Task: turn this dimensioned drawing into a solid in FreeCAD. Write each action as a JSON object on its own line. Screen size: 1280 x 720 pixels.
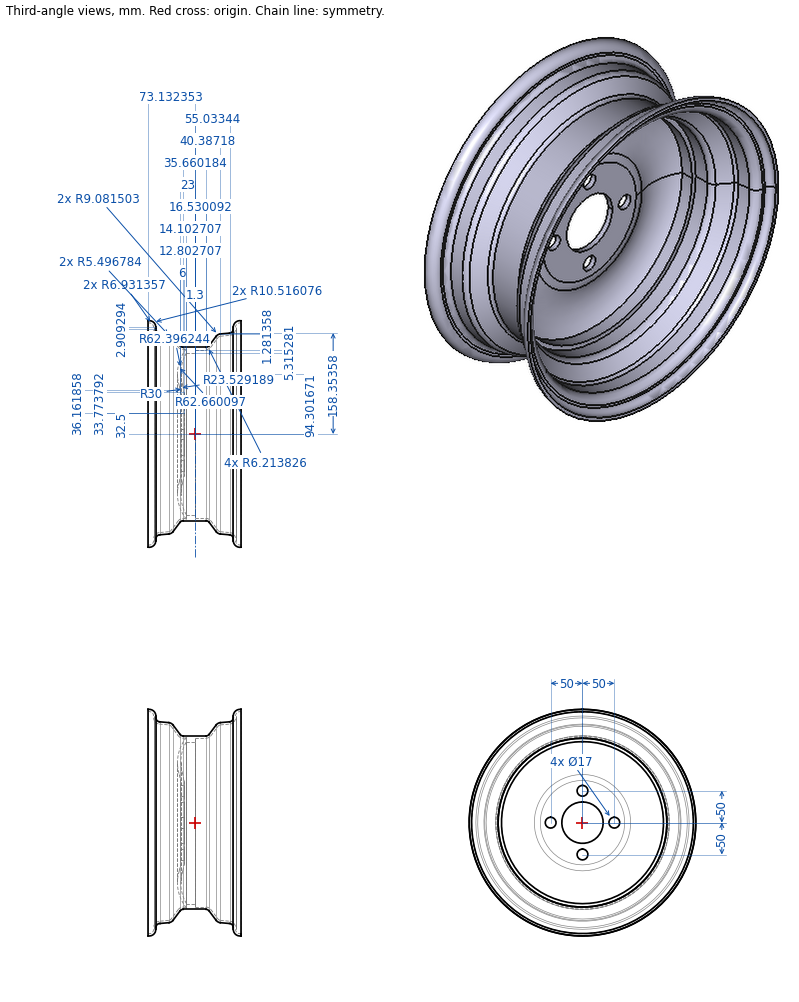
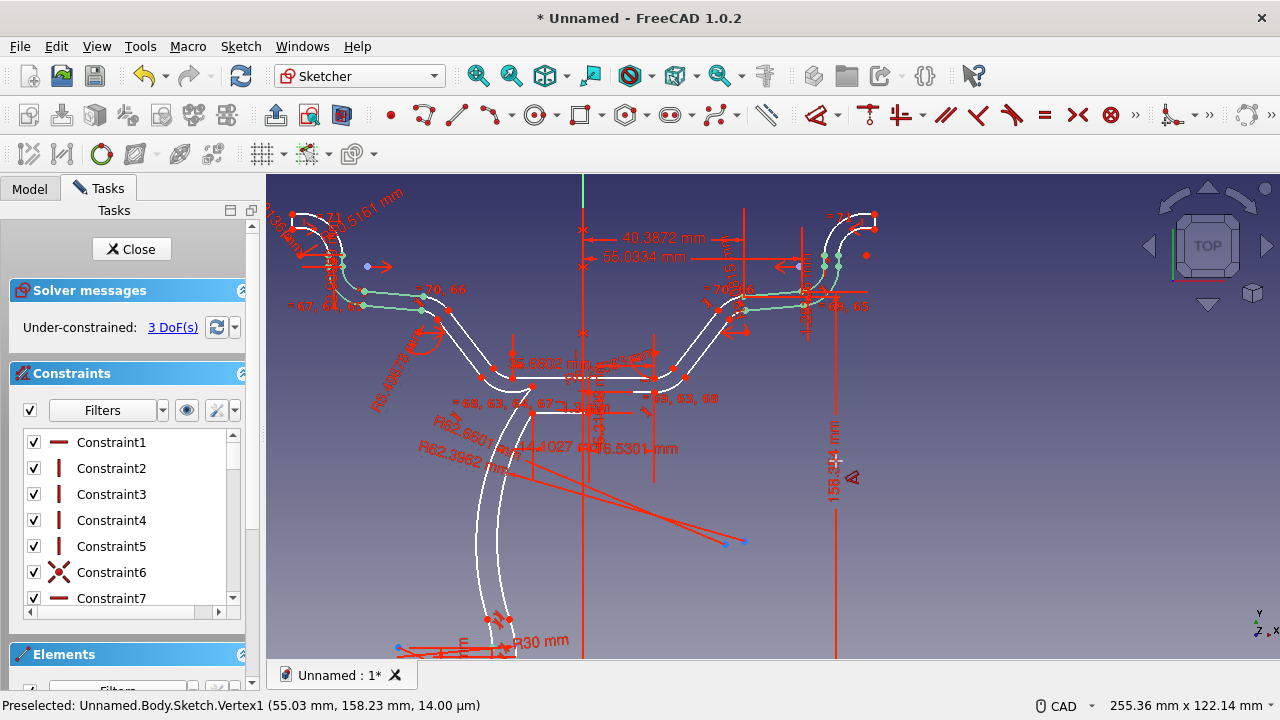
{"action": "scroll", "coordinate": [803, 293], "scroll_direction": "down", "scroll_amount": 4}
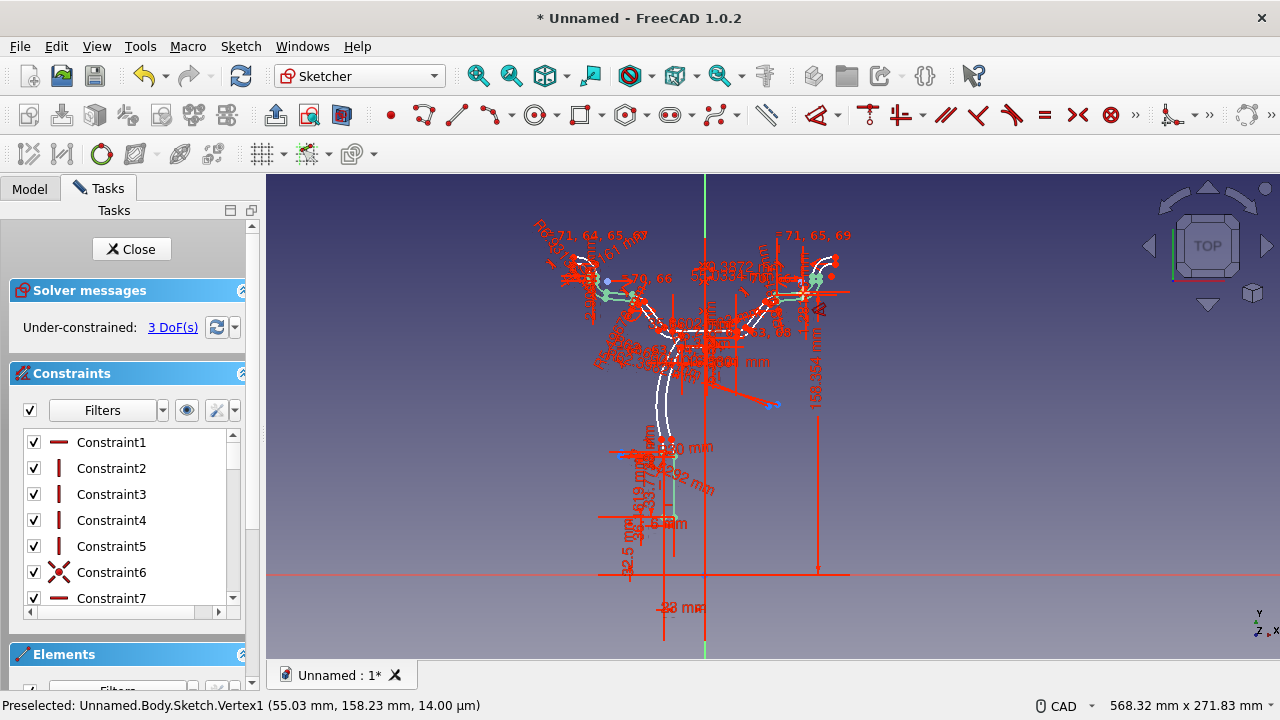
{"action": "scroll", "coordinate": [574, 258], "scroll_direction": "up", "scroll_amount": 4}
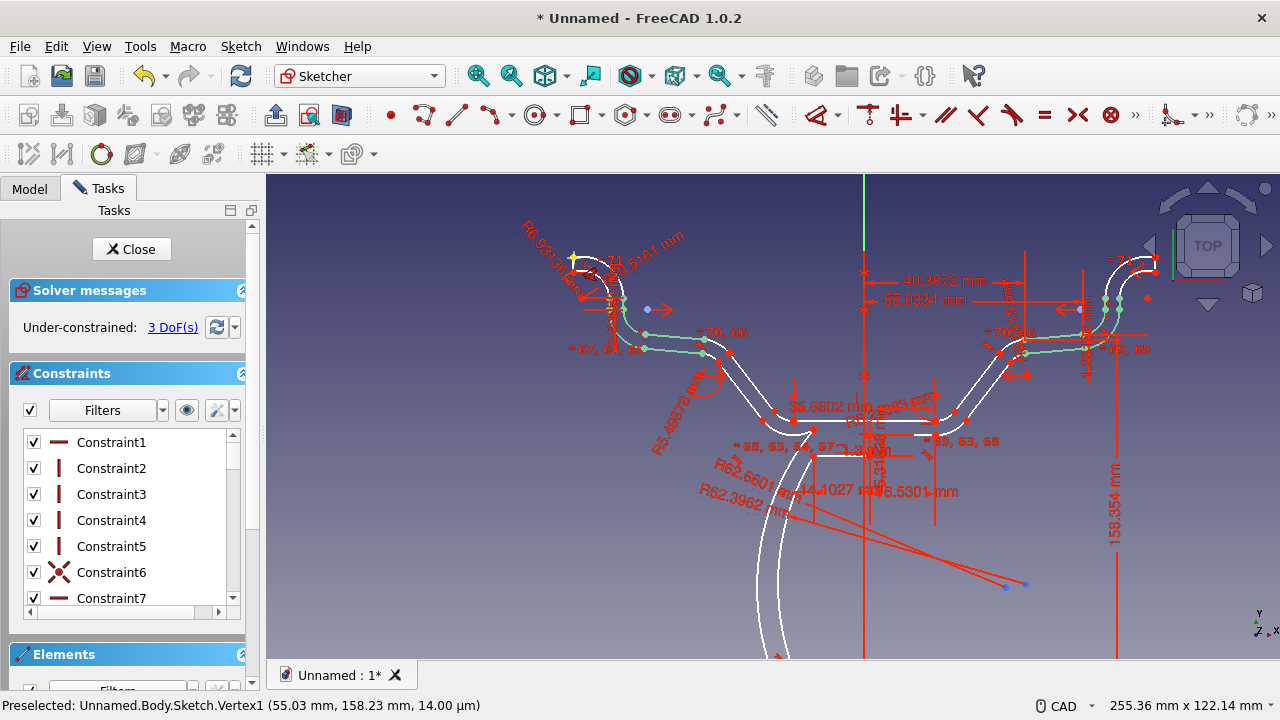
{"action": "left_click", "coordinate": [573, 257]}
{"action": "left_click", "coordinate": [719, 223]}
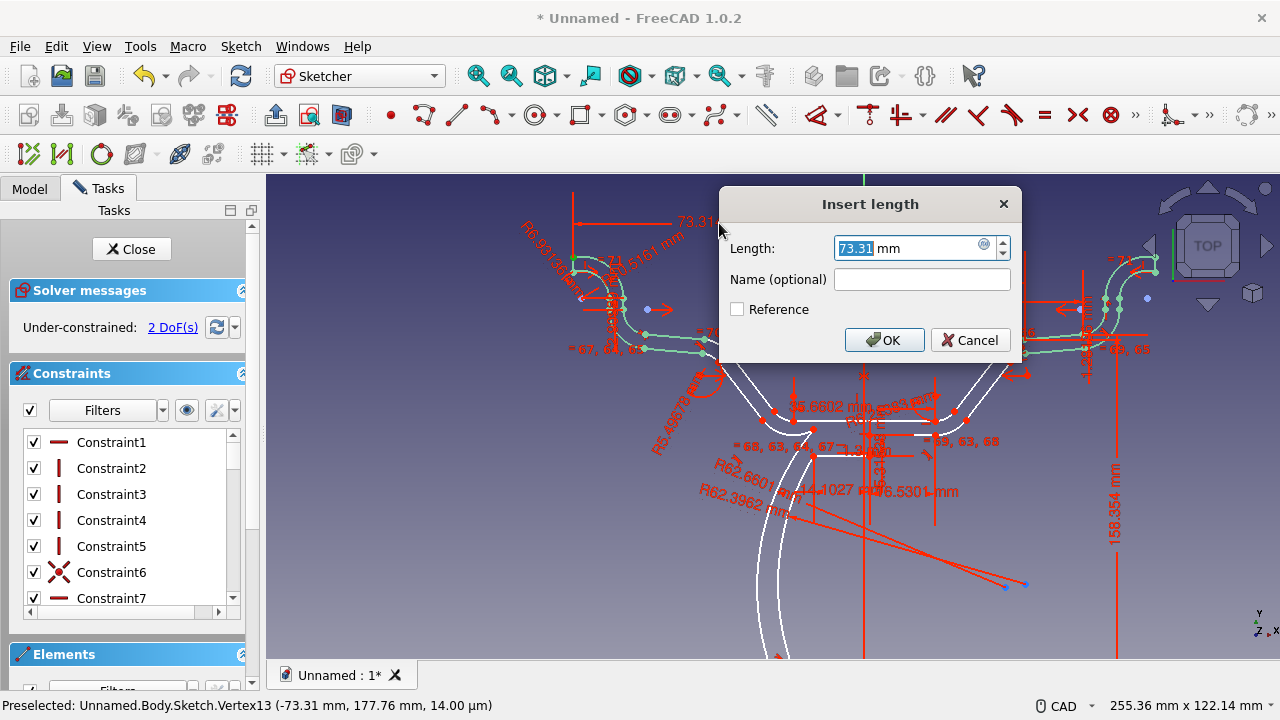
{"action": "type", "text": "73.132353"}
{"action": "key", "text": "Return"}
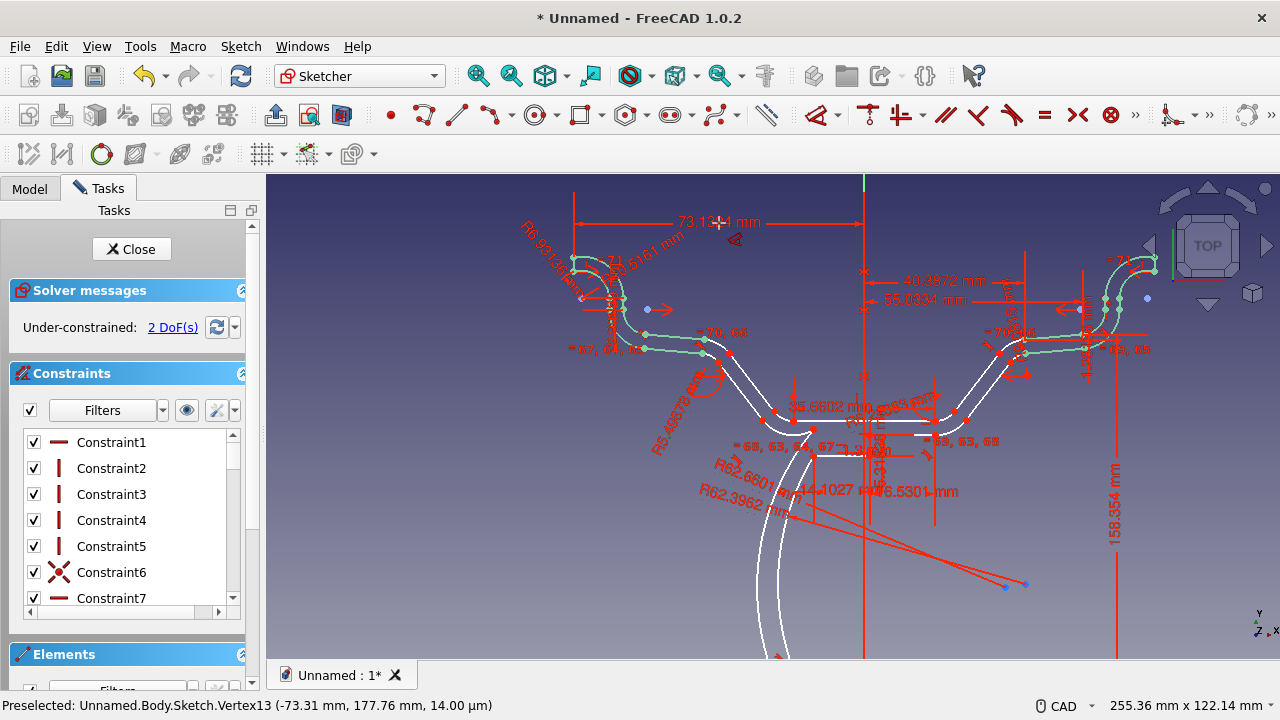
{"action": "left_click", "coordinate": [814, 430]}
{"action": "left_click", "coordinate": [839, 372]}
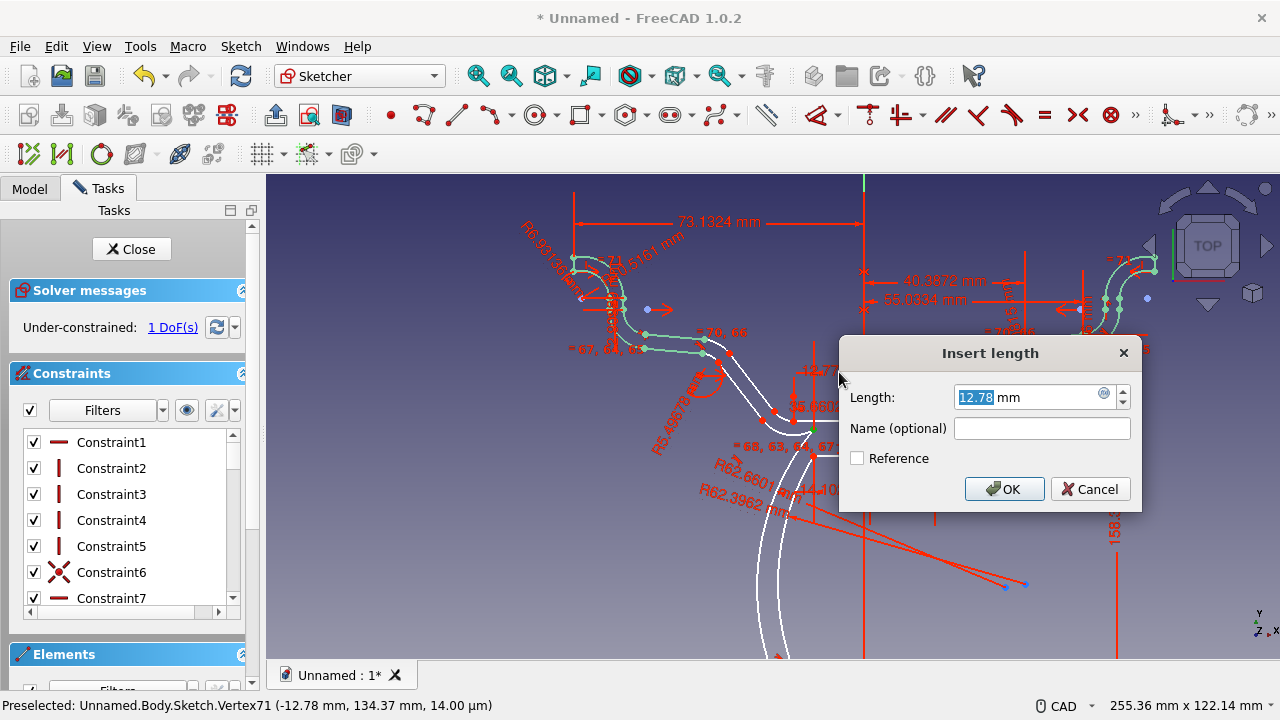
{"action": "type", "text": "12.802707"}
{"action": "key", "text": "Return"}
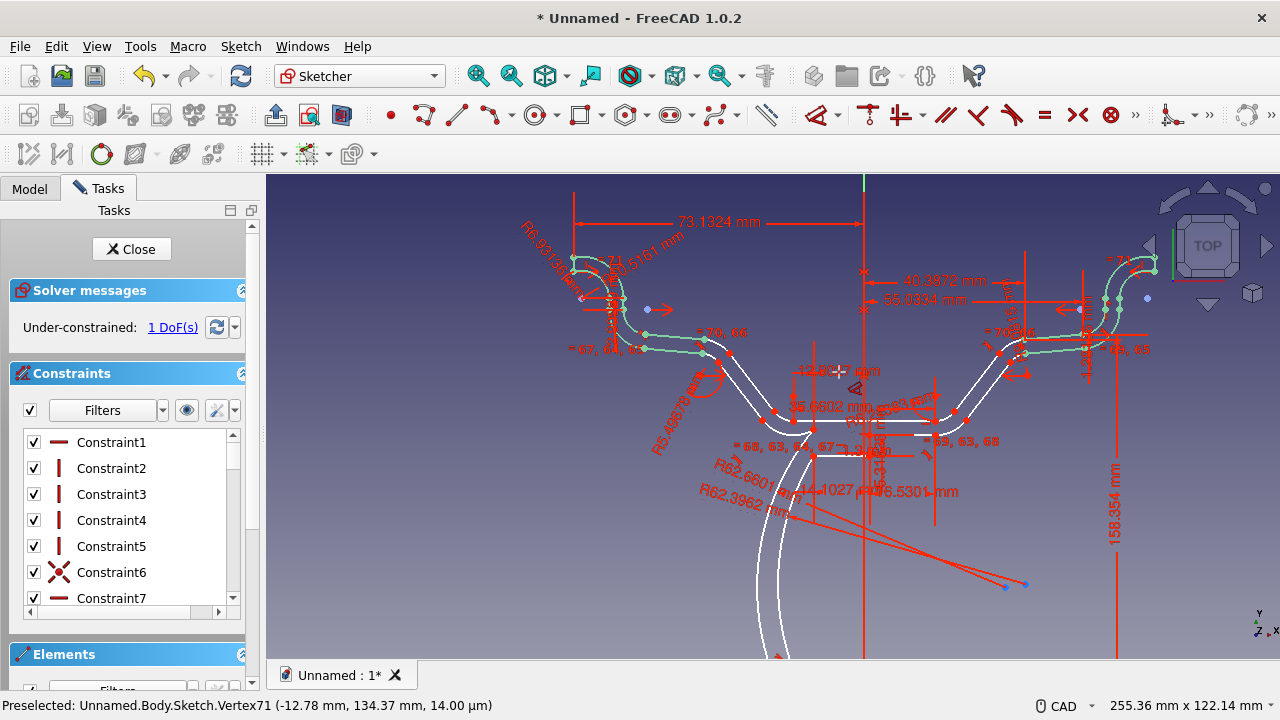
{"action": "left_click", "coordinate": [1006, 588]}
{"action": "left_click", "coordinate": [1040, 609]}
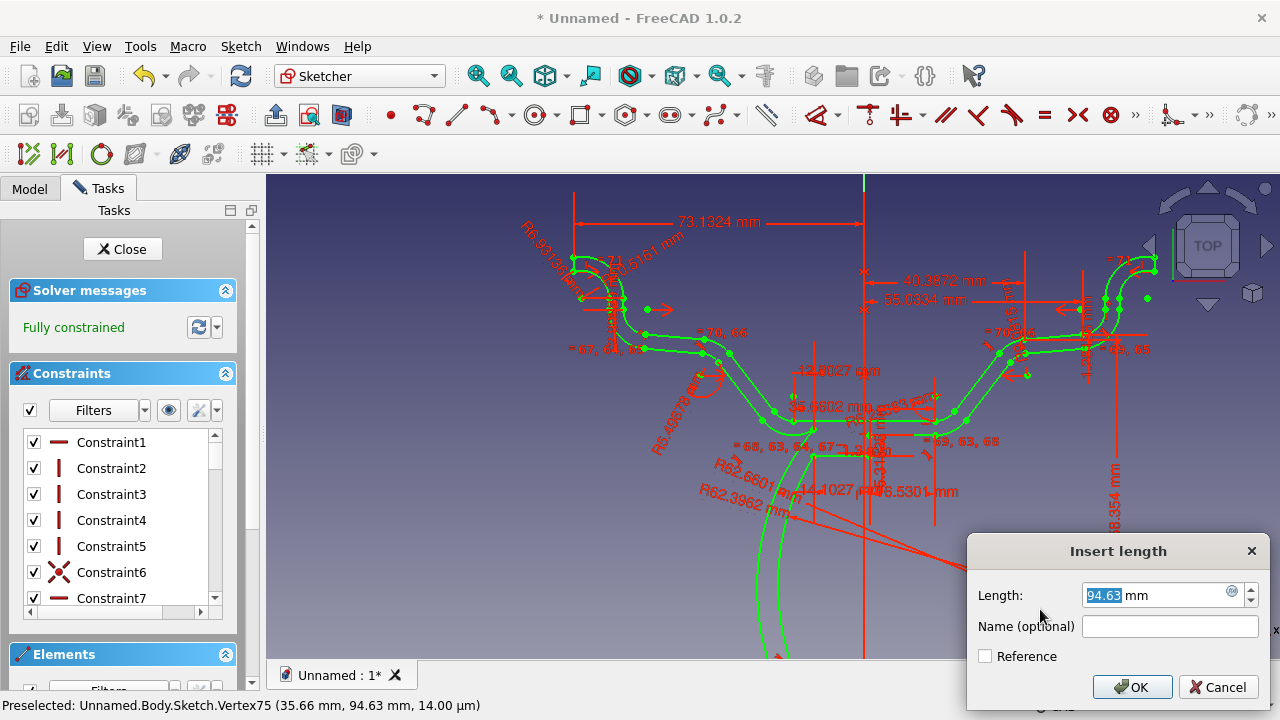
{"action": "type", "text": "94.301671"}
{"action": "key", "text": "Return"}
{"action": "key", "text": "Escape"}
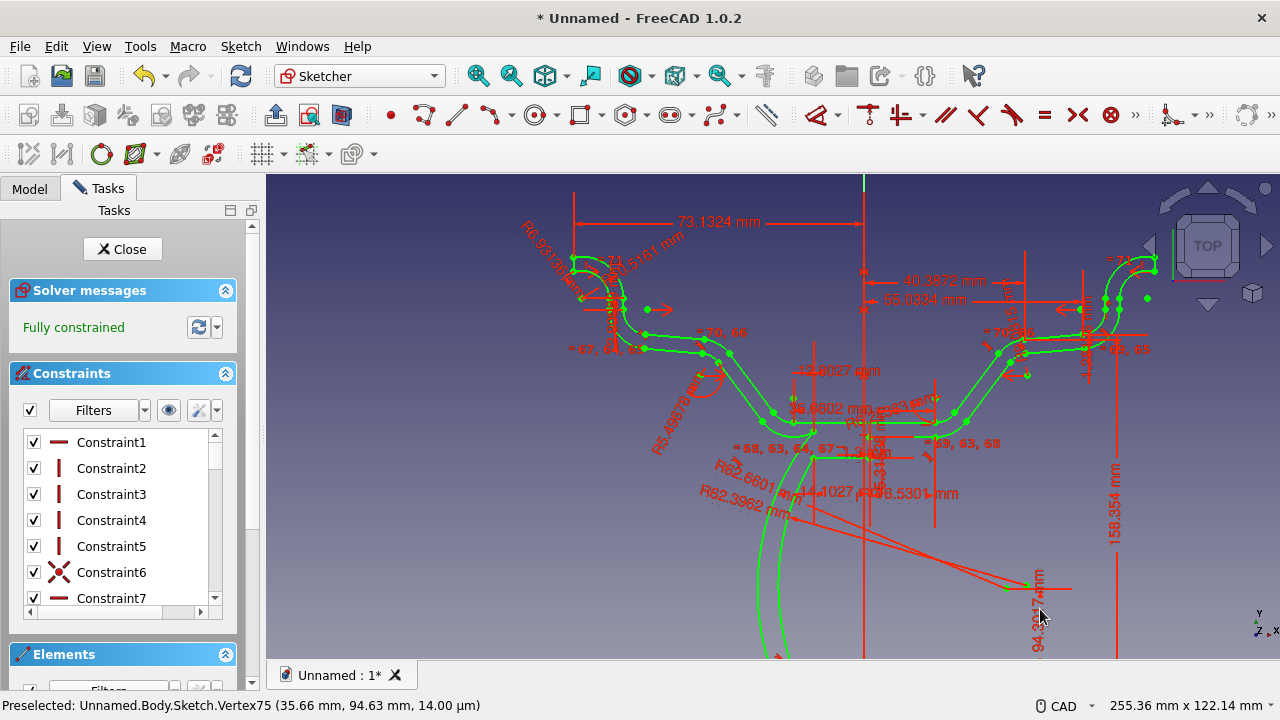
{"action": "left_click", "coordinate": [123, 249]}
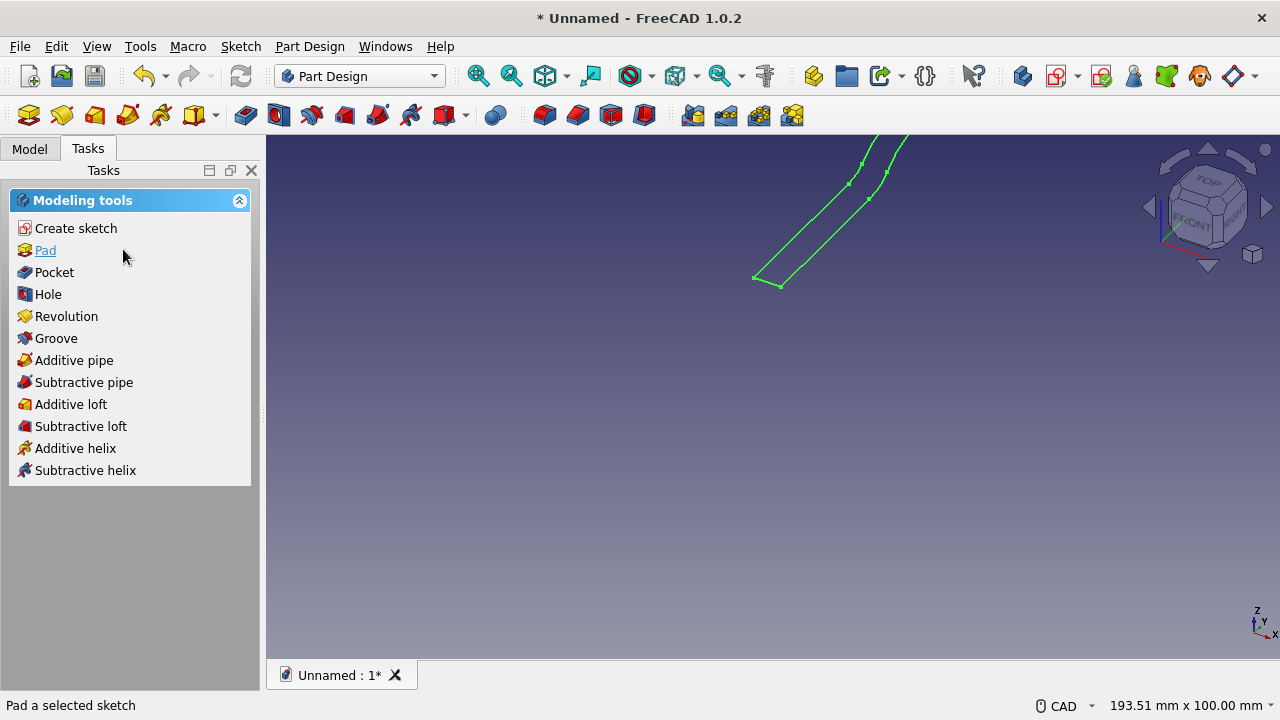
{"action": "left_click", "coordinate": [62, 116]}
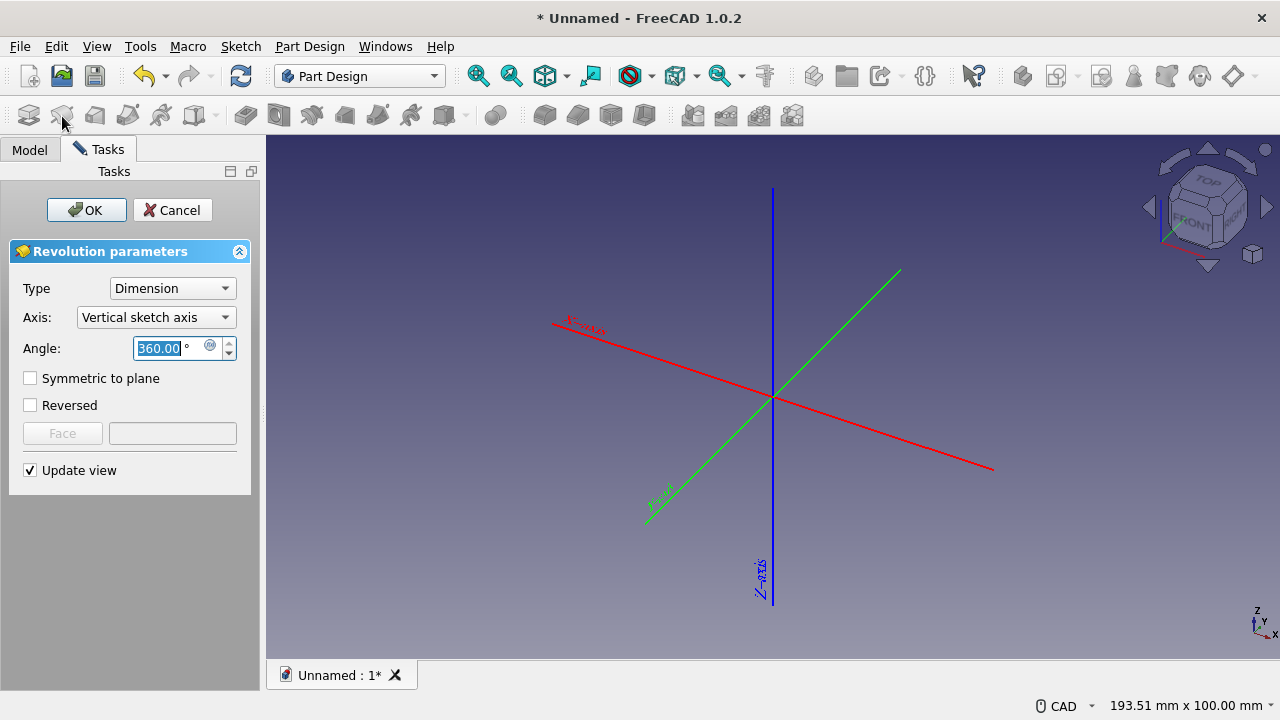
{"action": "left_click", "coordinate": [157, 318]}